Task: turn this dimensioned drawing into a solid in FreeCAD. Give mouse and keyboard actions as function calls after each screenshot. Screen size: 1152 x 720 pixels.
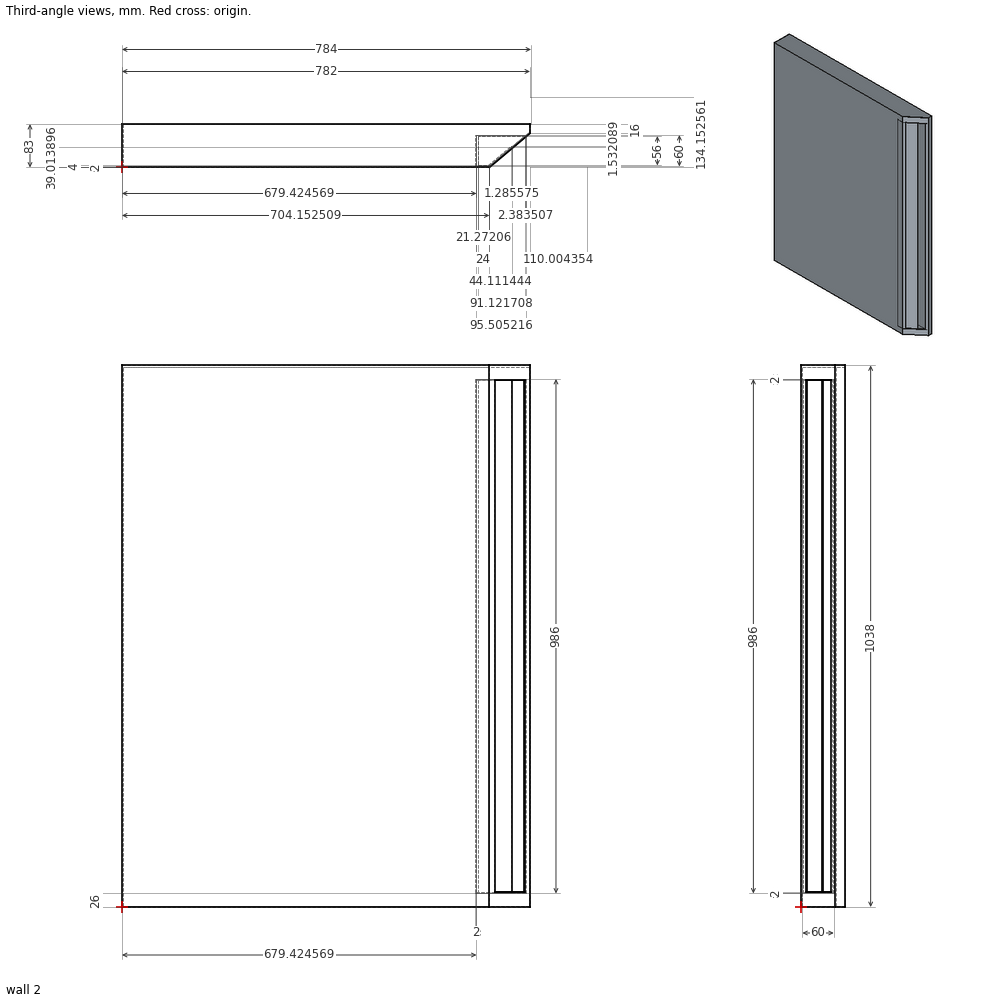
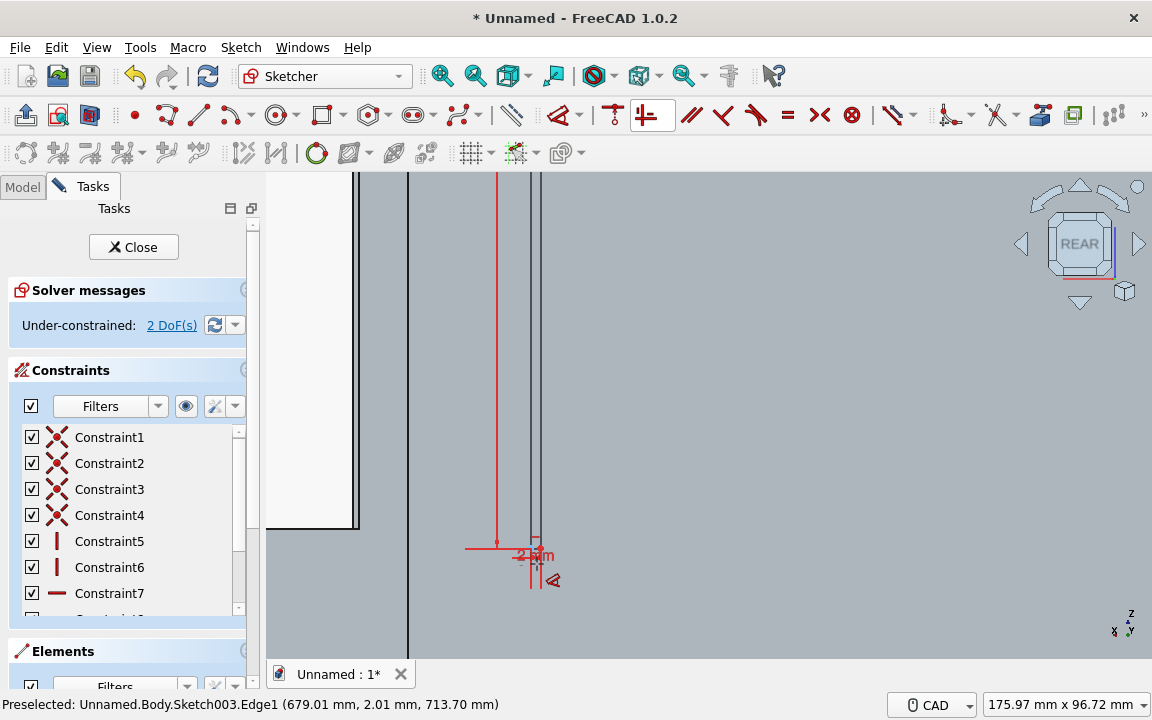
click(531, 549)
click(497, 590)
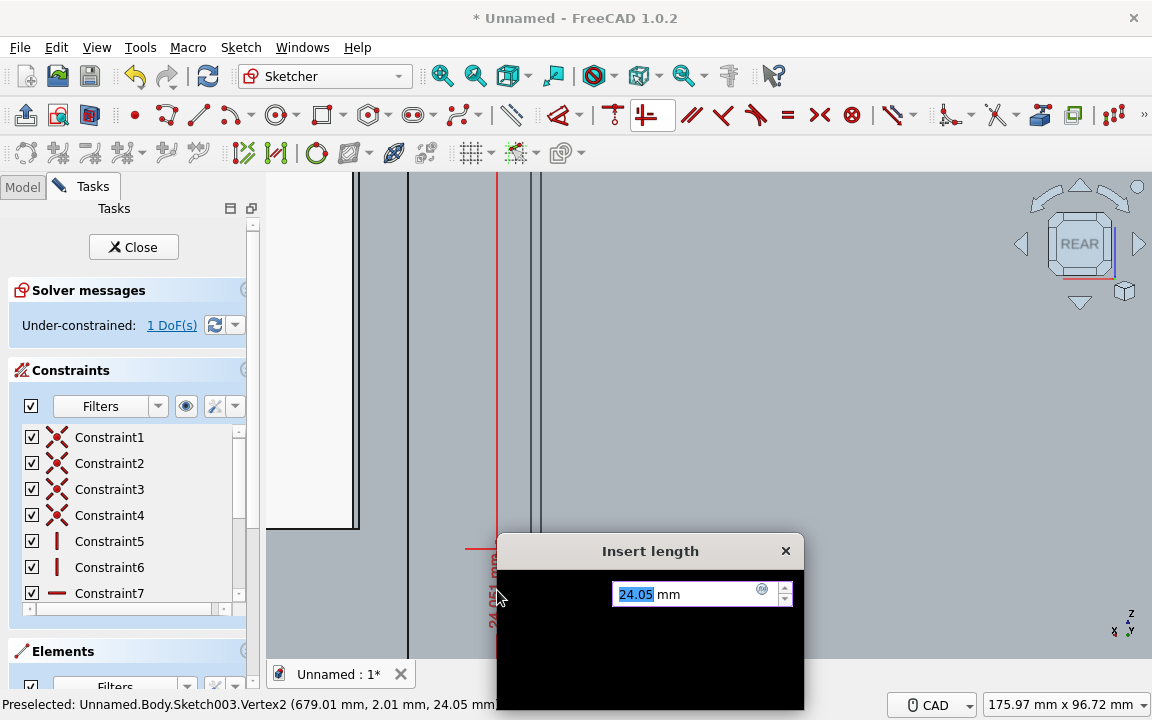
text(26)
key(Return)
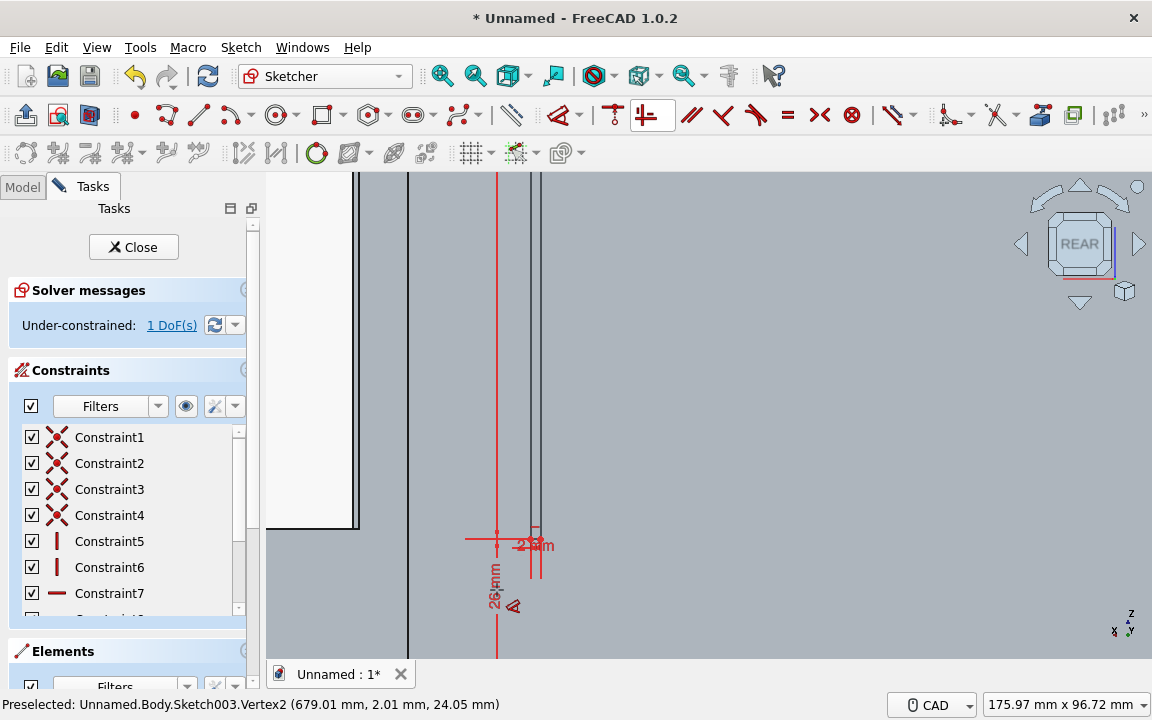
scroll(537, 564, down, 14)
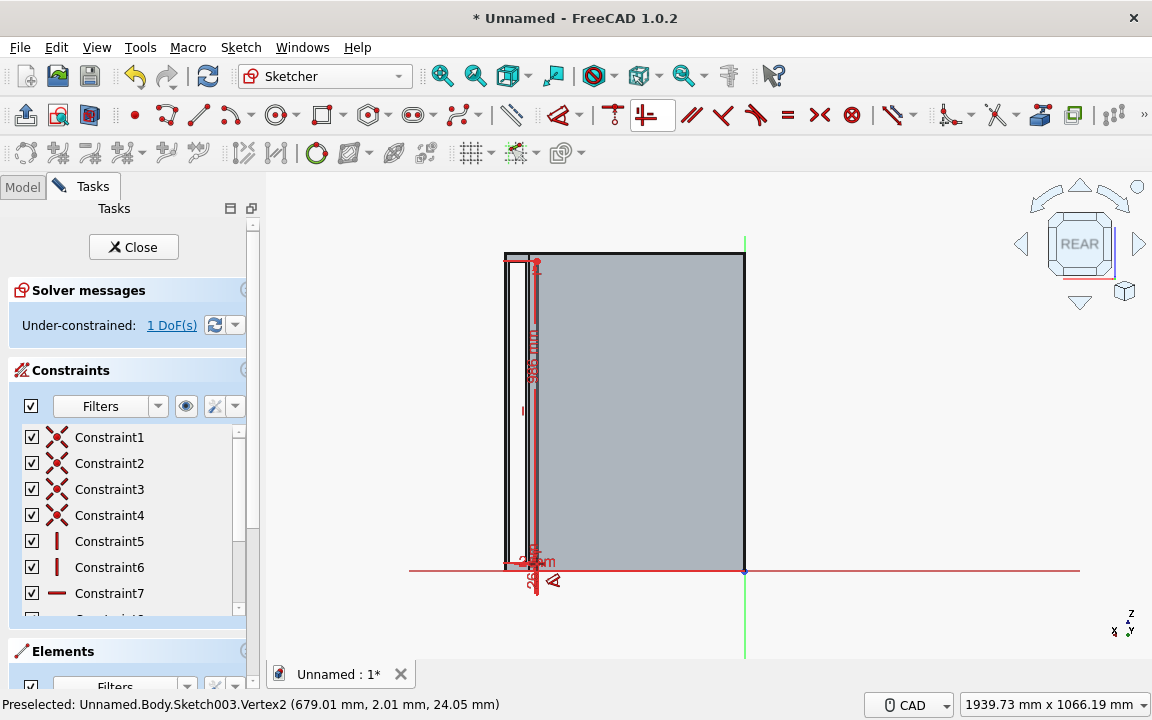
scroll(537, 261, up, 14)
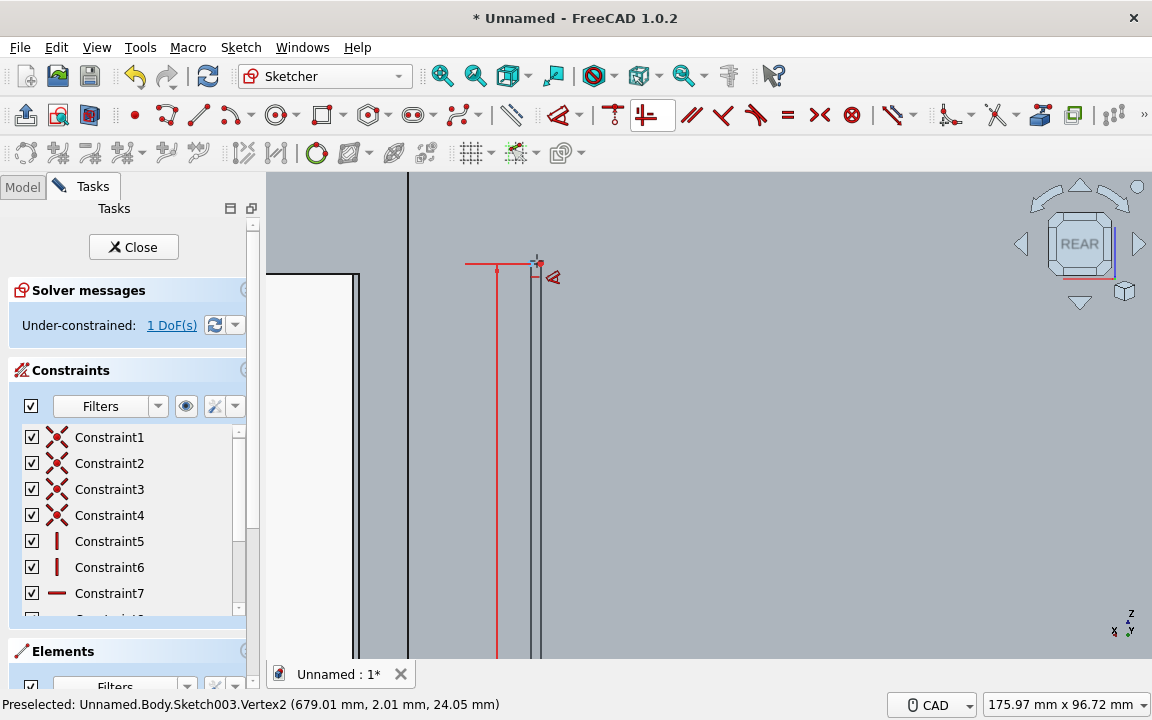
click(531, 264)
click(759, 230)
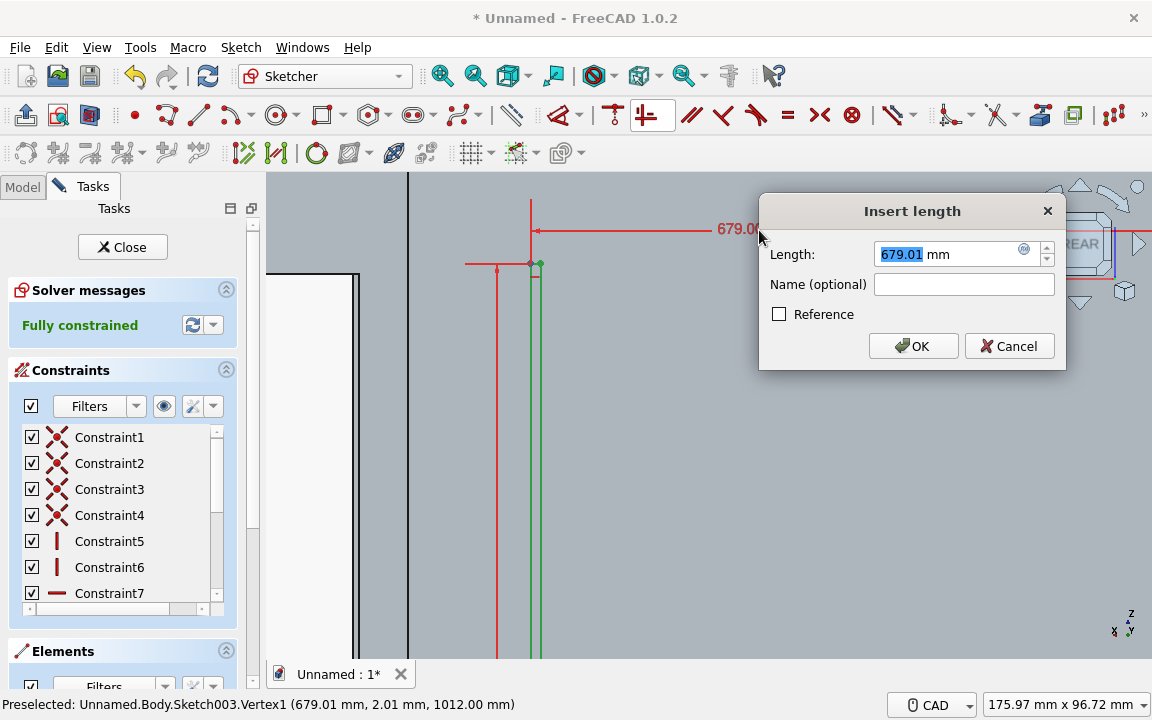
text(679.424569)
key(Return)
key(Escape)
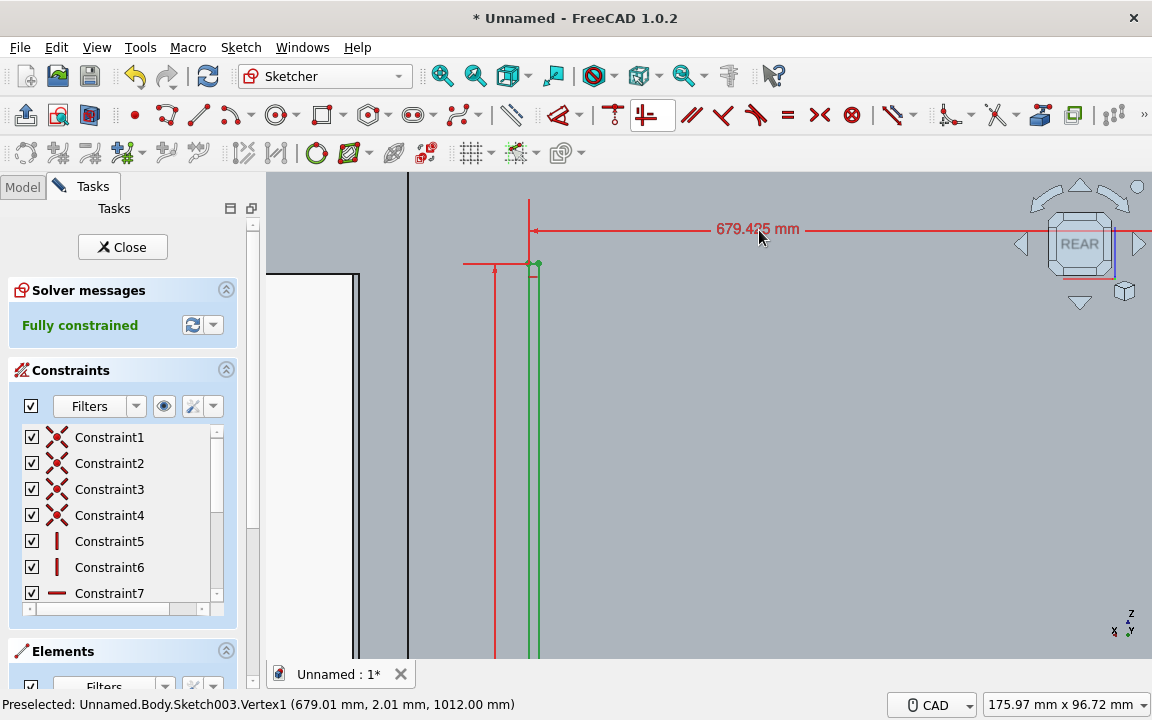
click(123, 247)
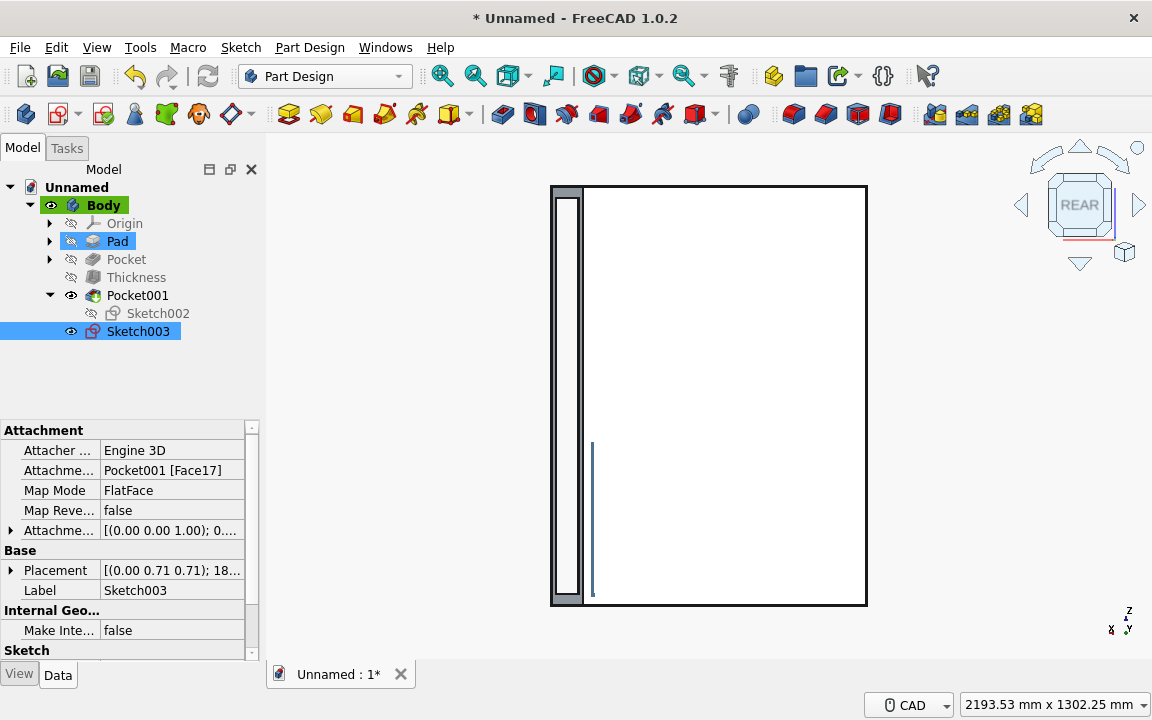
click(290, 114)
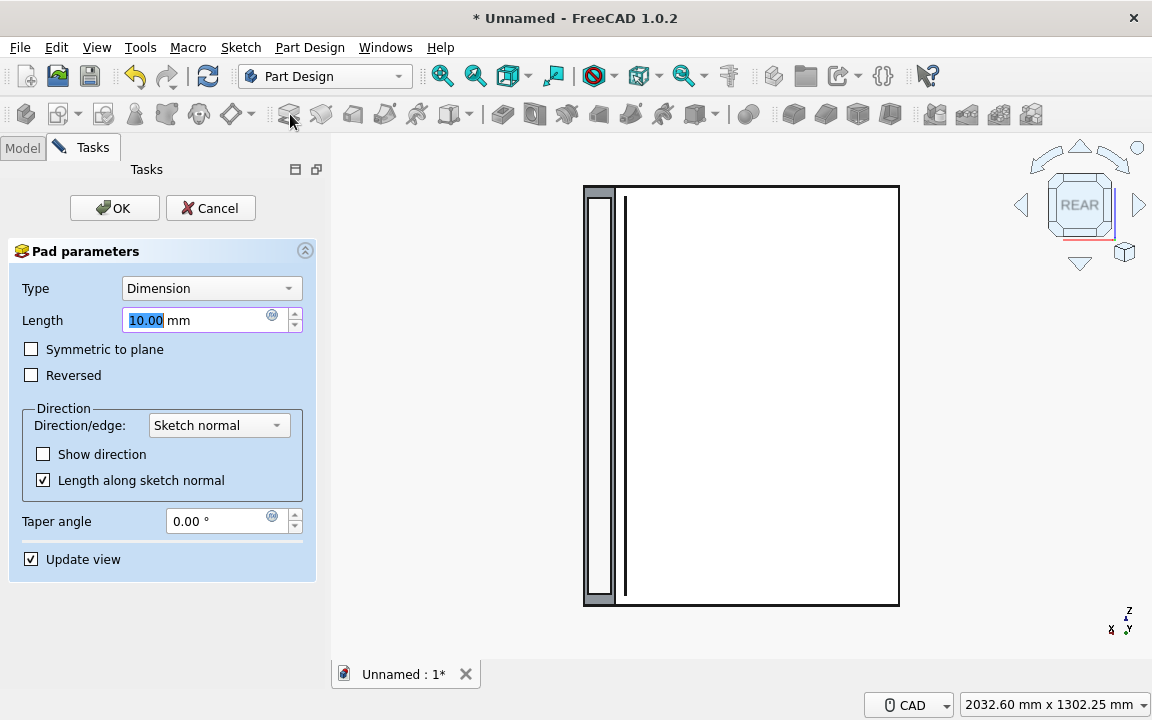
text(60)
key(Tab)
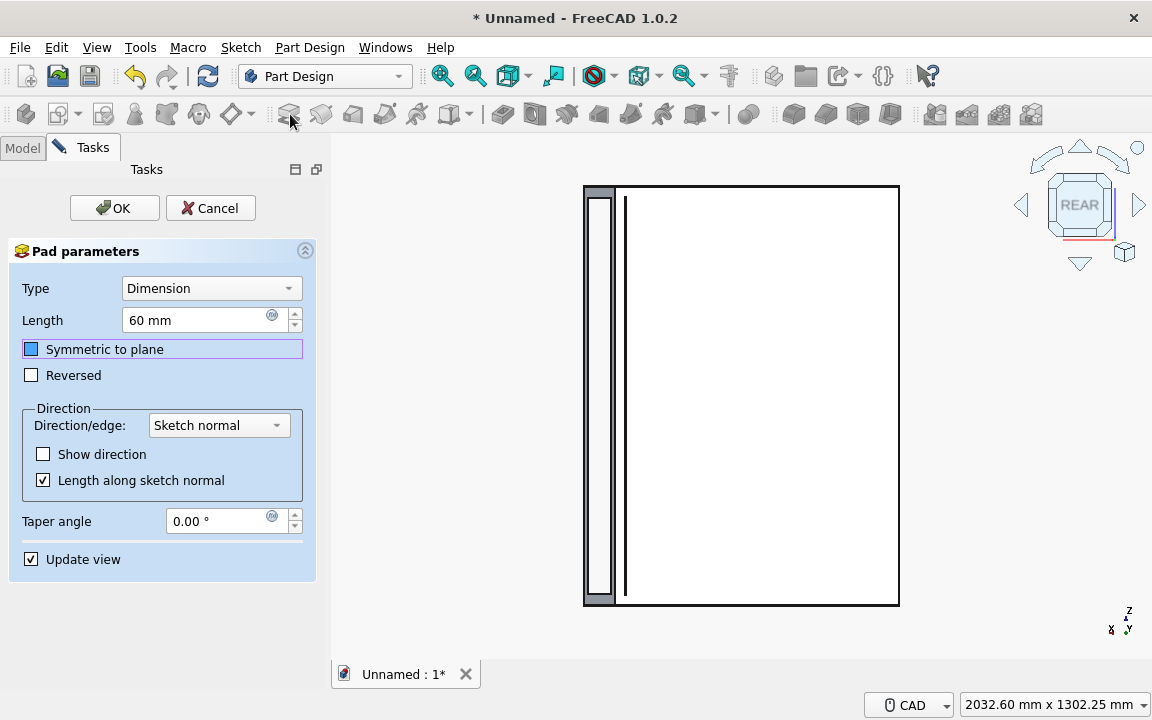
click(115, 208)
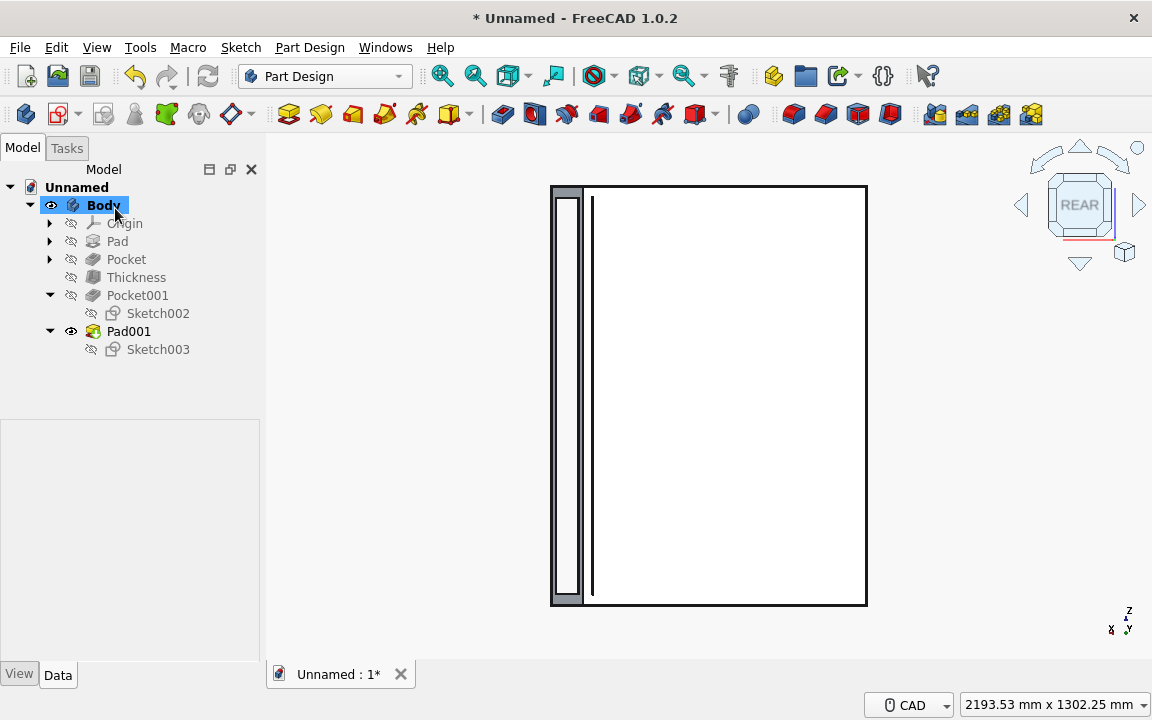
click(26, 114)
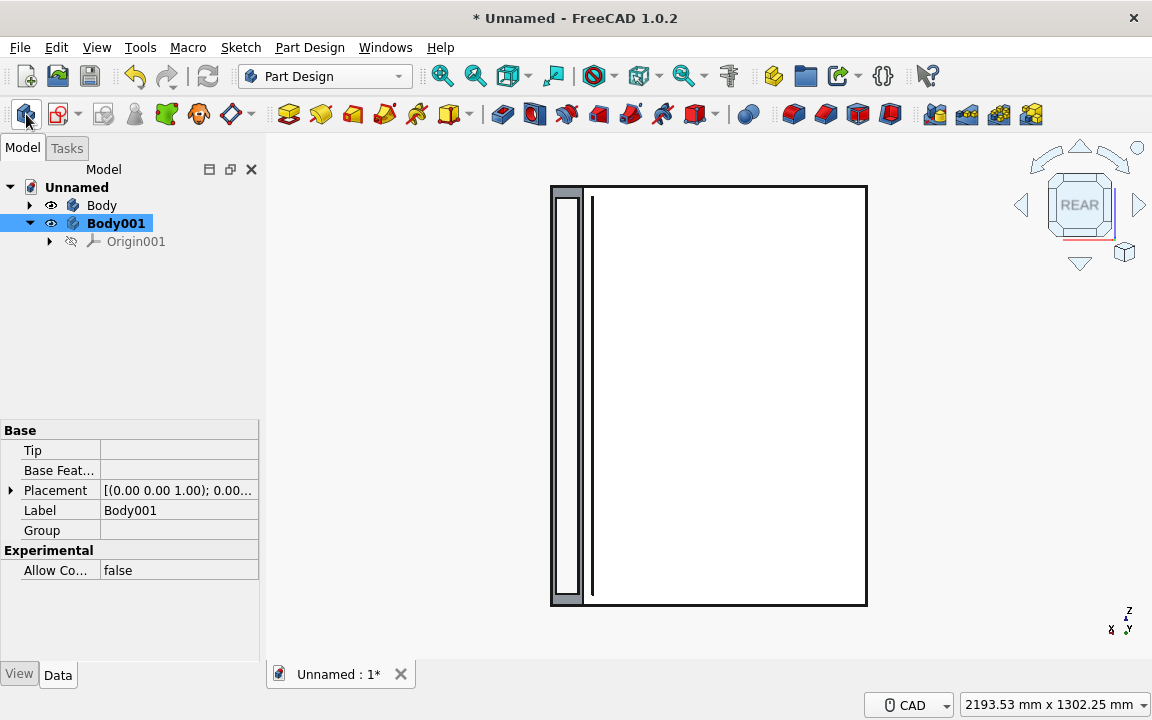
click(50, 241)